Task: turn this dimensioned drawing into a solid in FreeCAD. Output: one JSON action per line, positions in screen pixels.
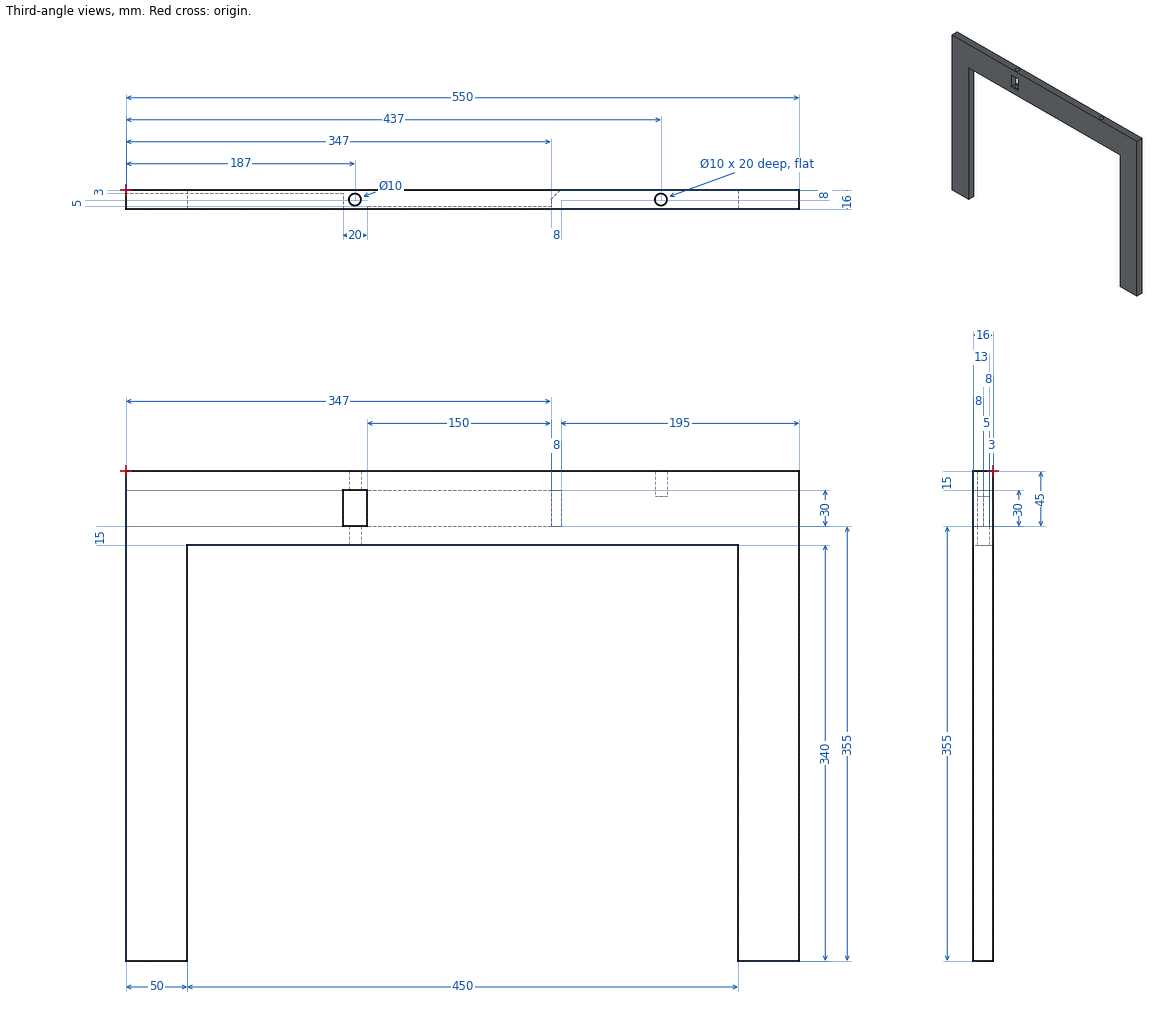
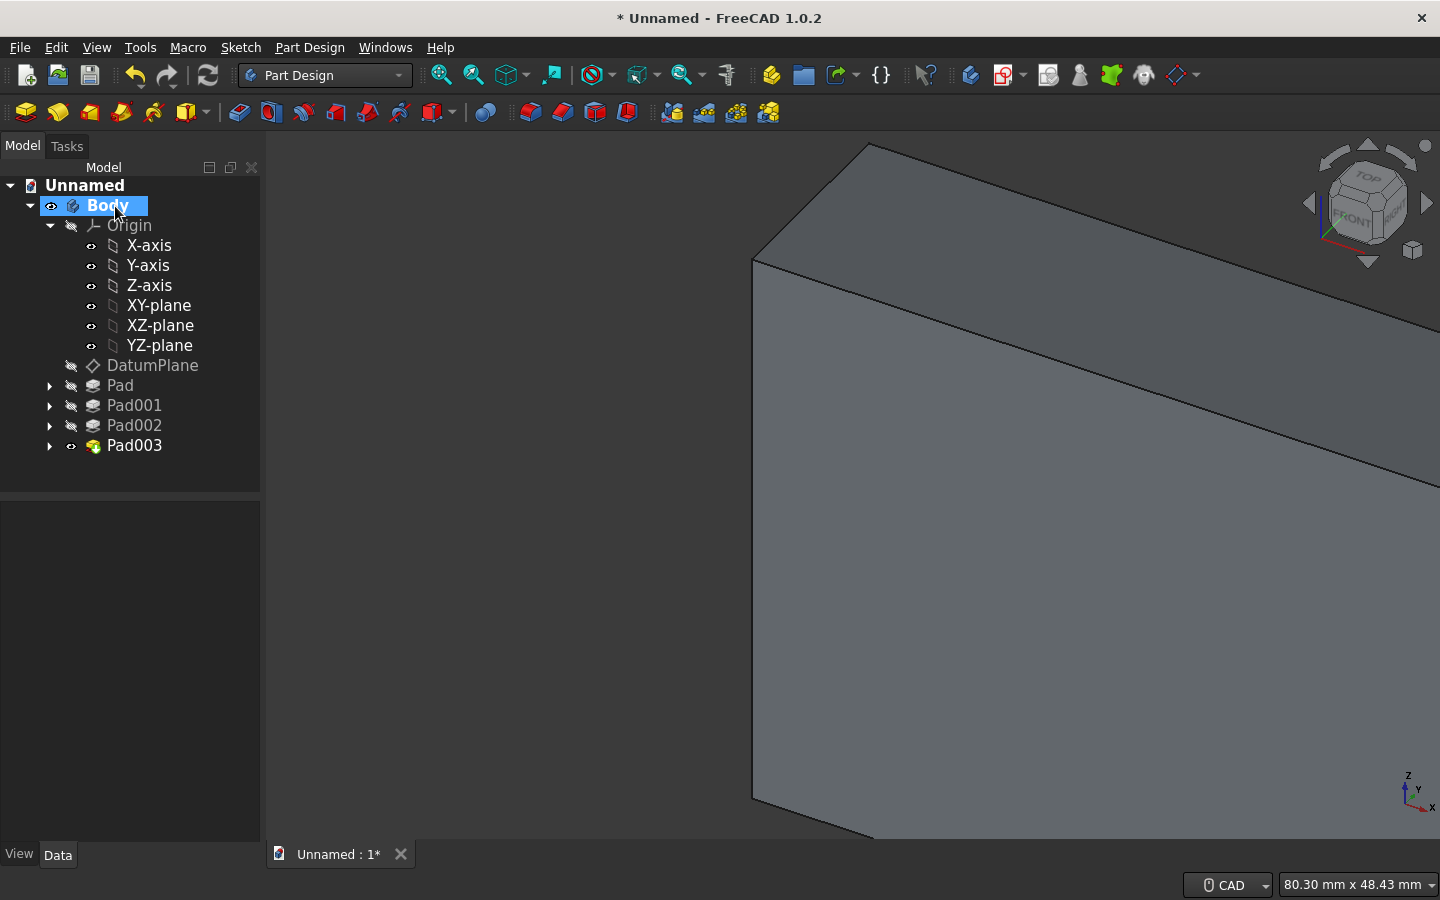
{"action": "left_click", "coordinate": [442, 76]}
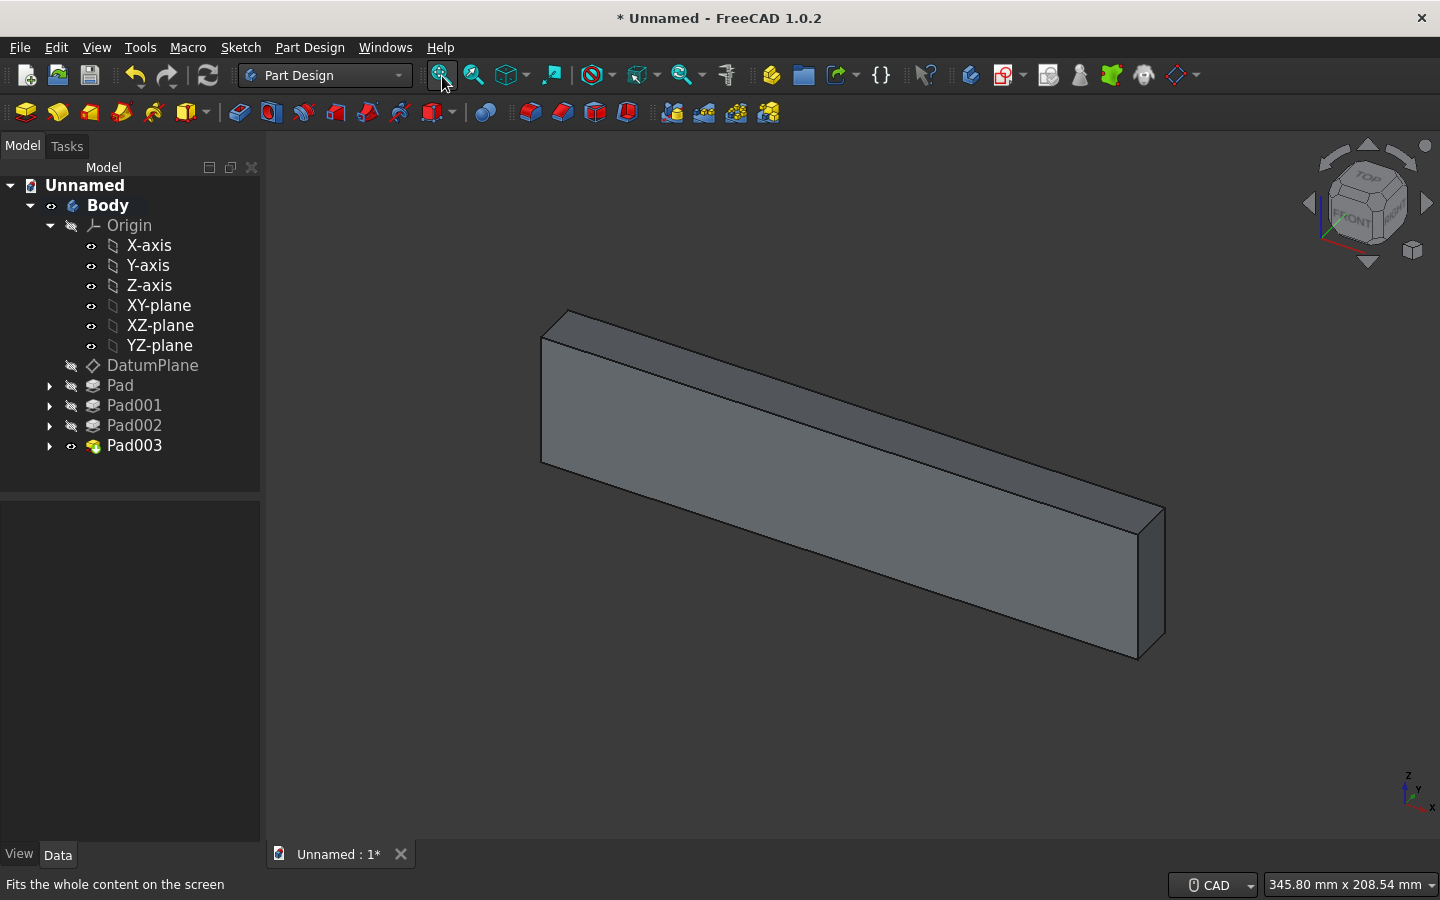
{"action": "key", "text": "6"}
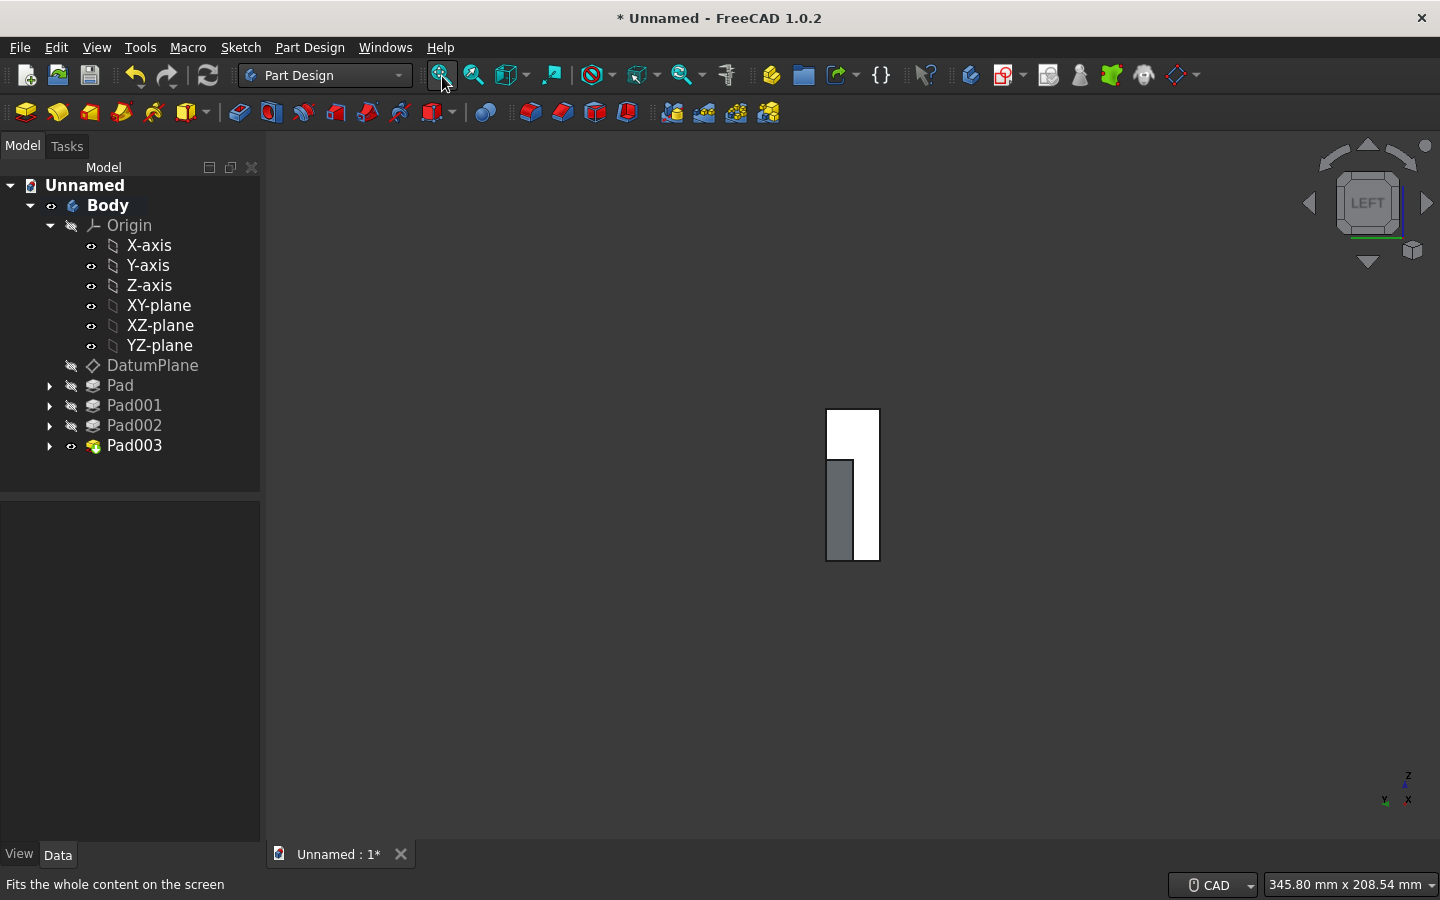
{"action": "left_click", "coordinate": [442, 76]}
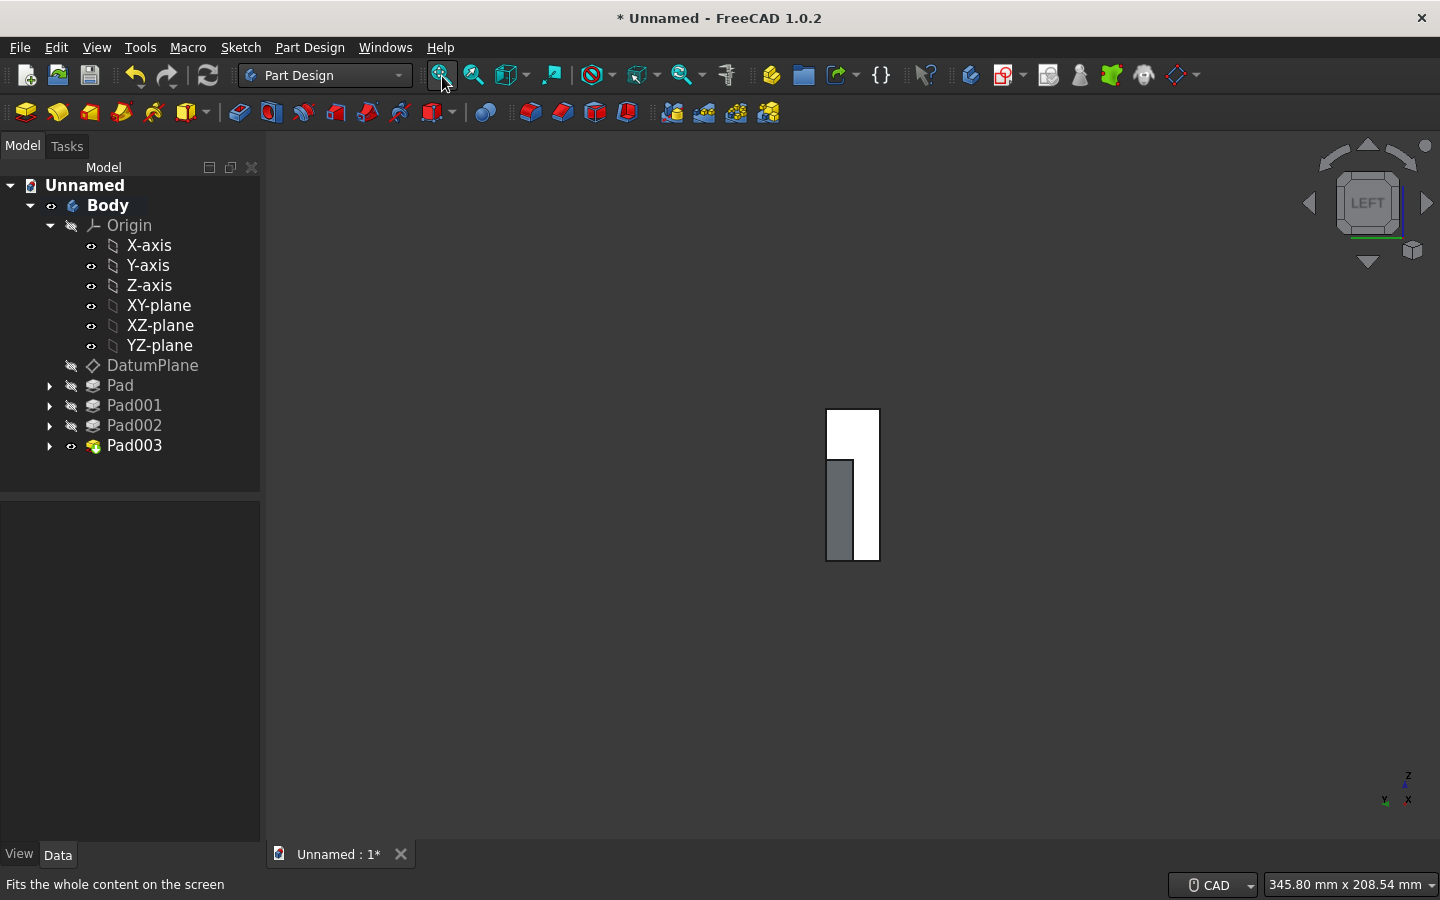
{"action": "left_click", "coordinate": [861, 440]}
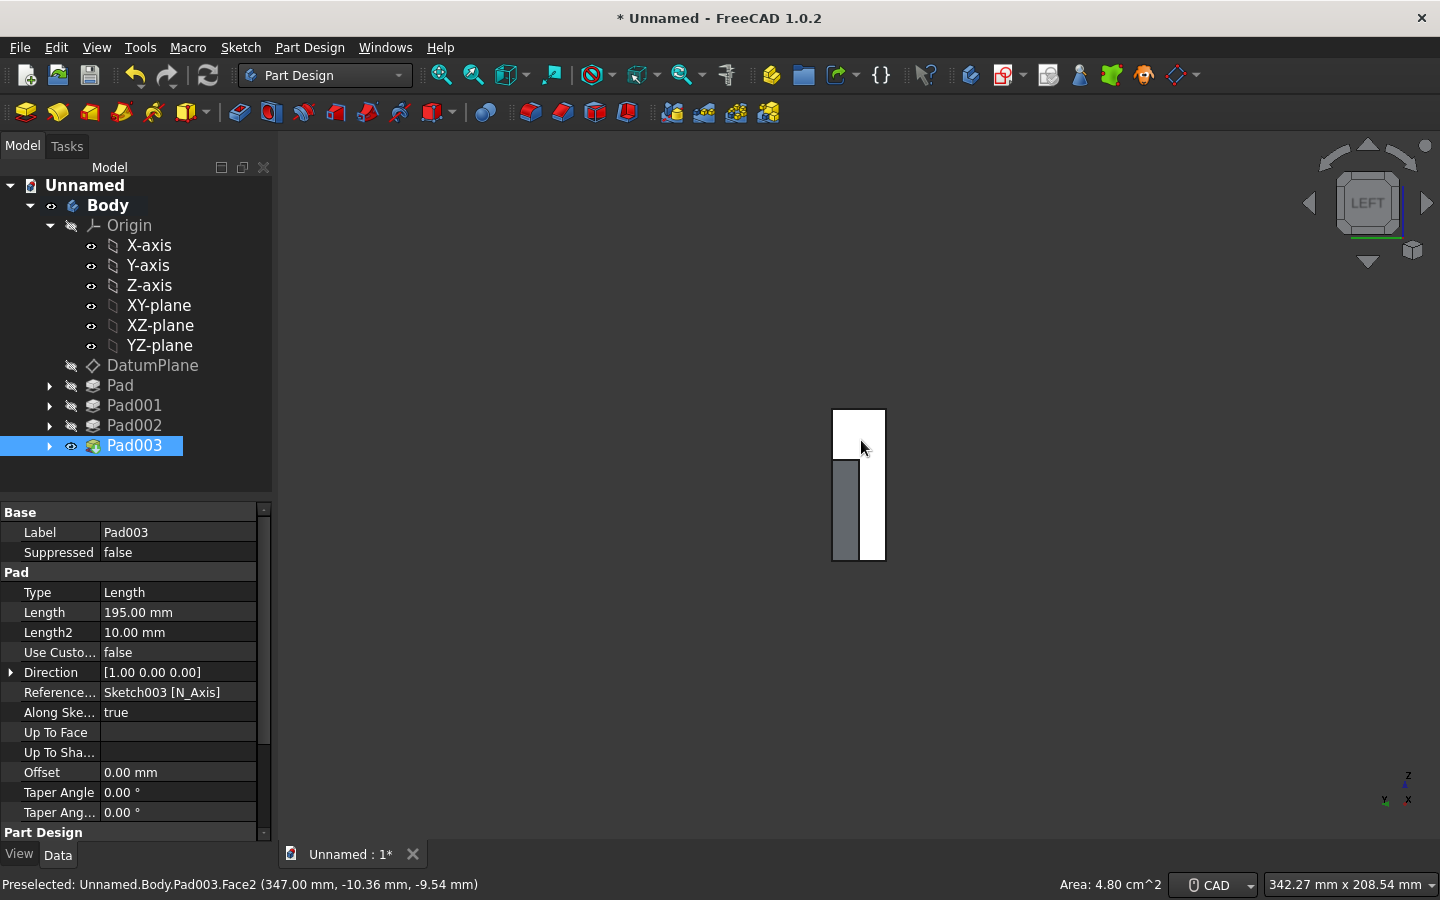
{"action": "left_click", "coordinate": [1004, 76]}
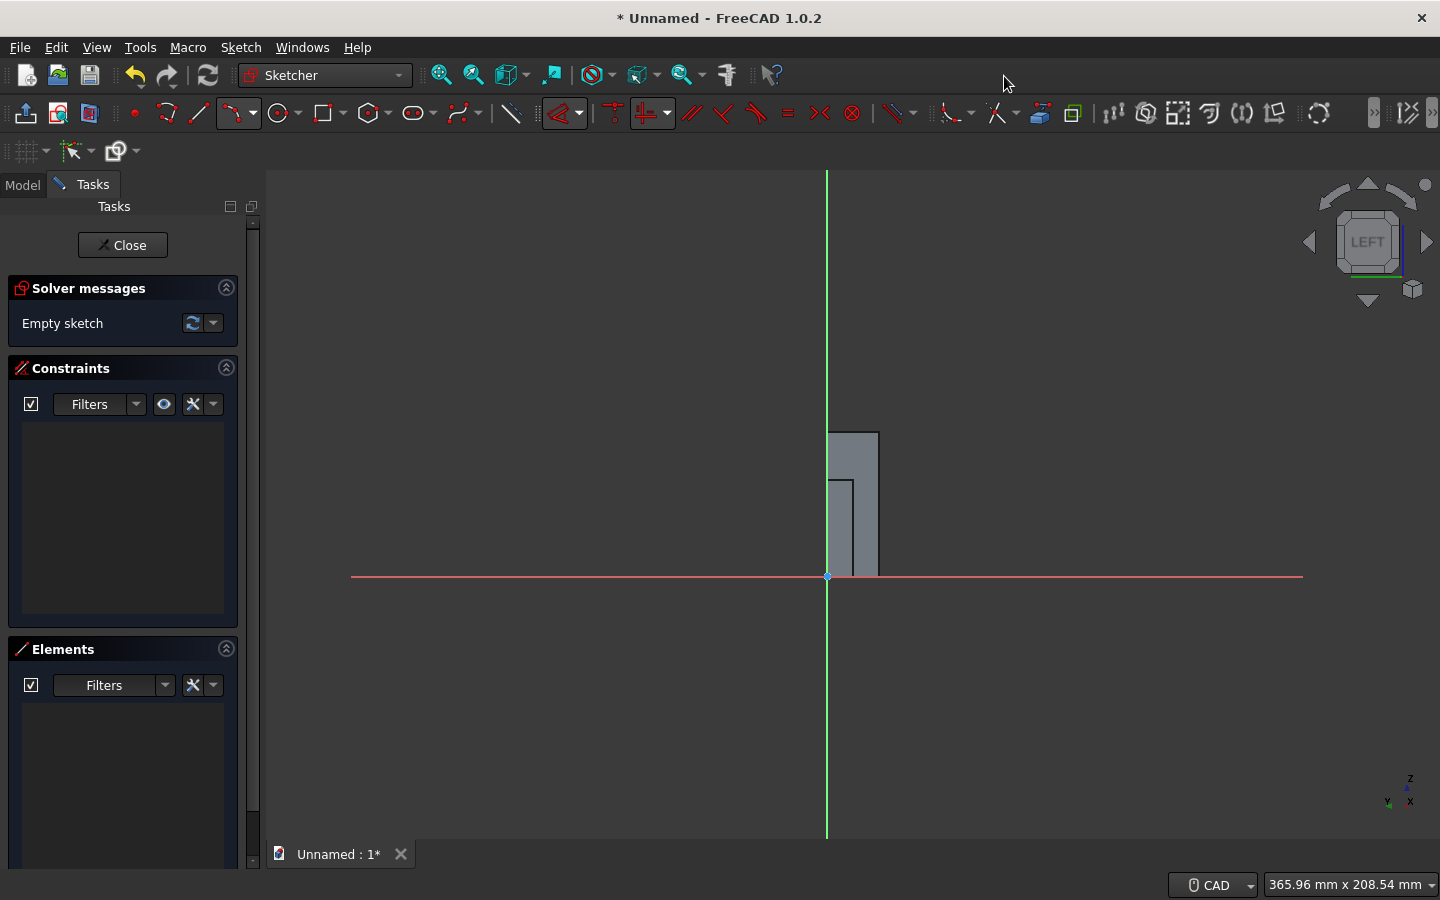
{"action": "scroll", "coordinate": [893, 504], "scroll_direction": "up", "scroll_amount": 5}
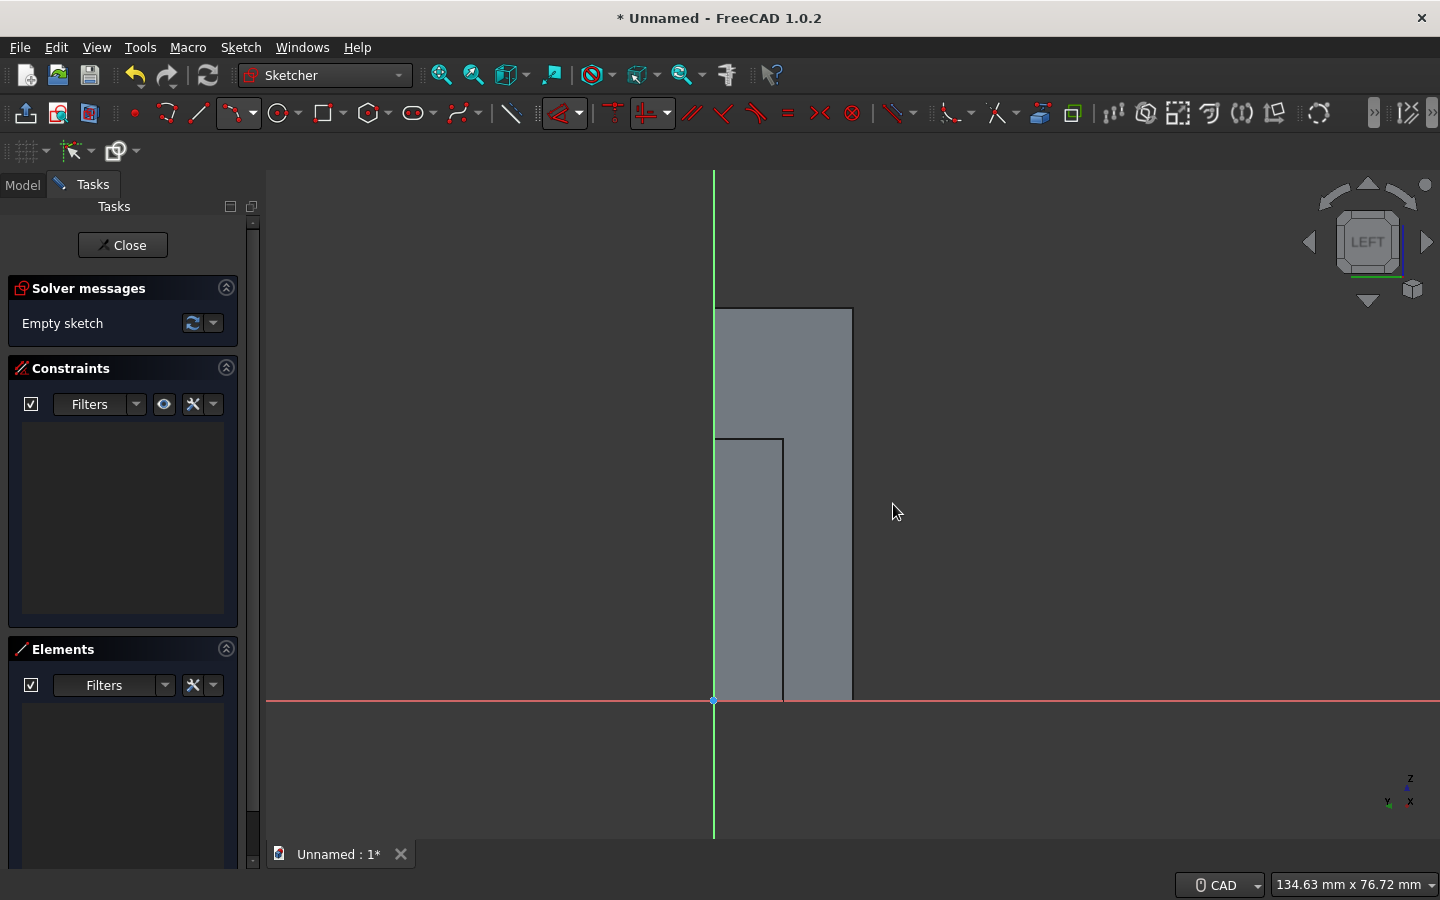
{"action": "left_click", "coordinate": [324, 114]}